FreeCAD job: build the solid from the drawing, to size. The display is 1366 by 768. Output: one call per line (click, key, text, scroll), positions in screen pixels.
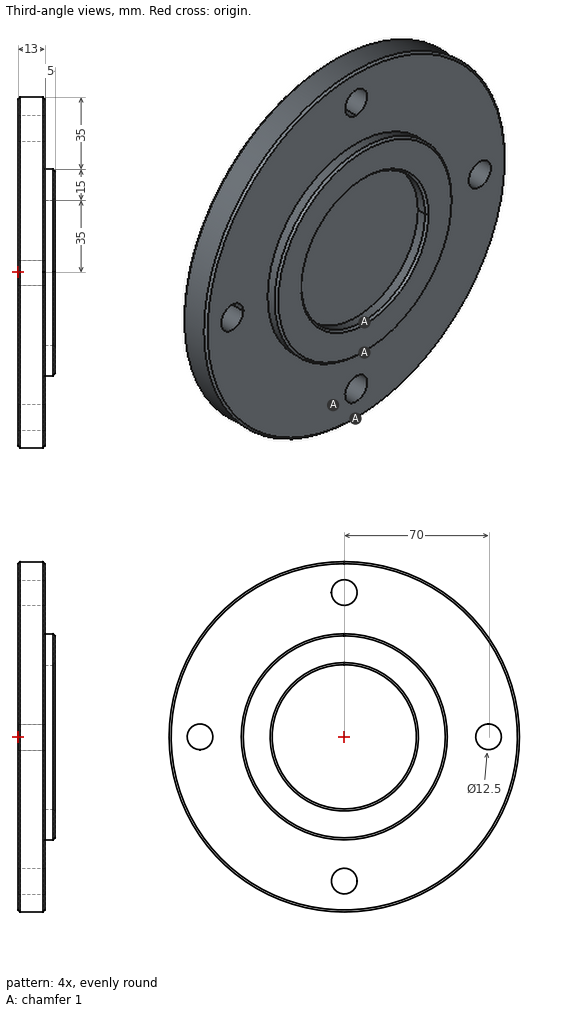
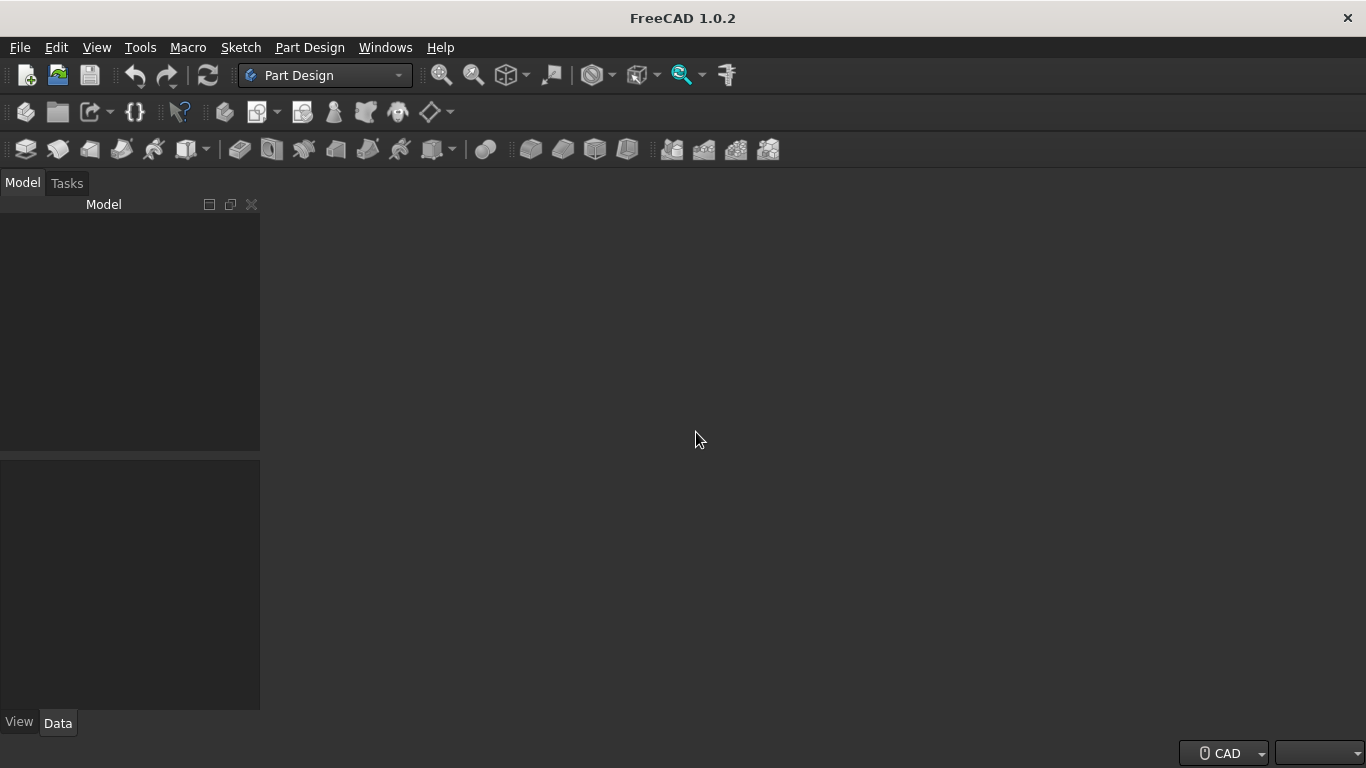
click(26, 76)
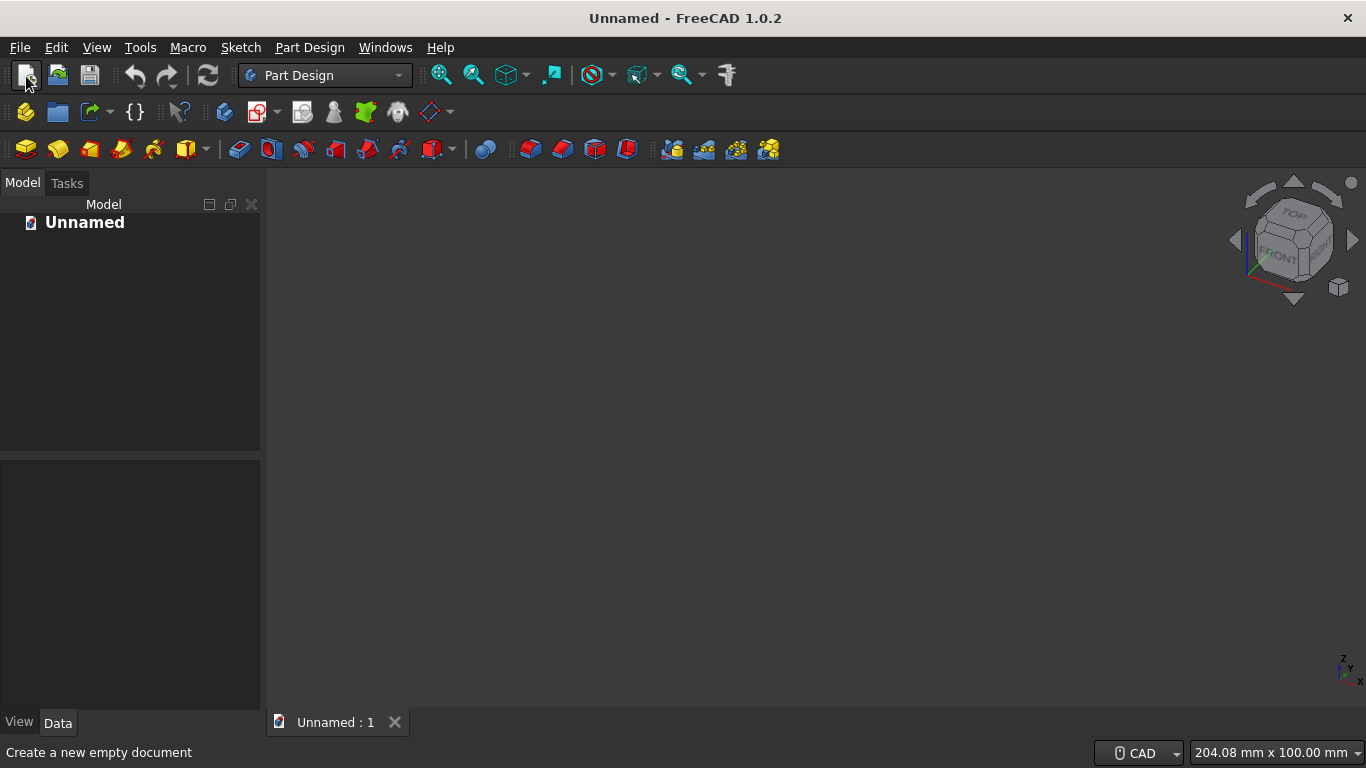
click(258, 112)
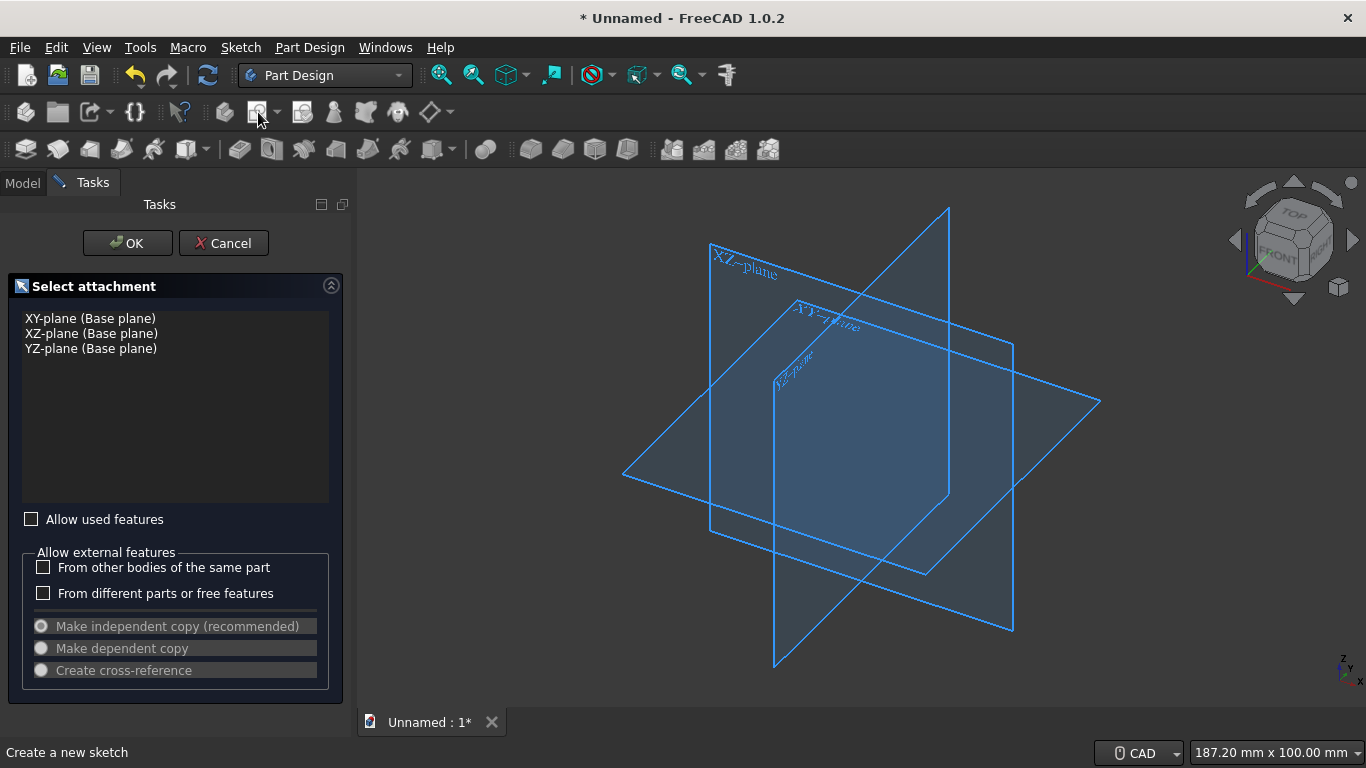
click(82, 318)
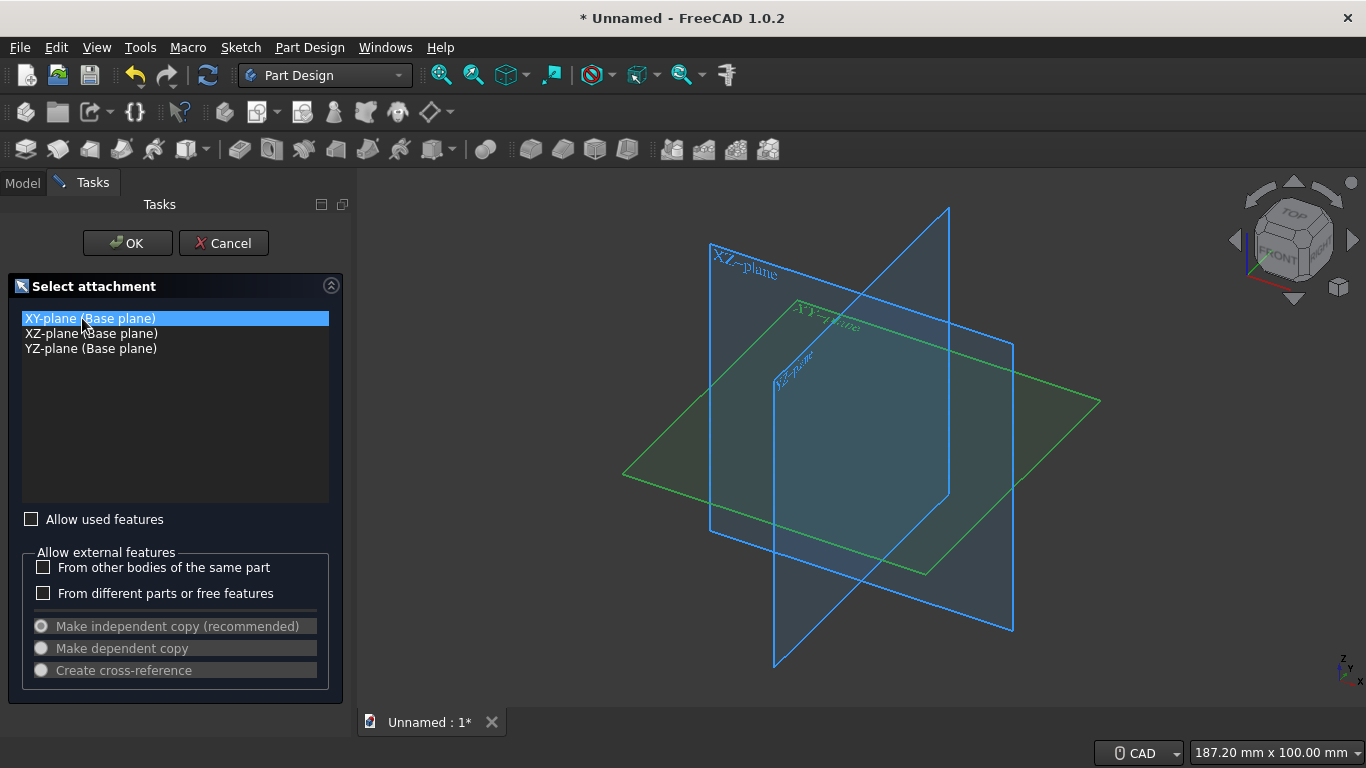
click(128, 243)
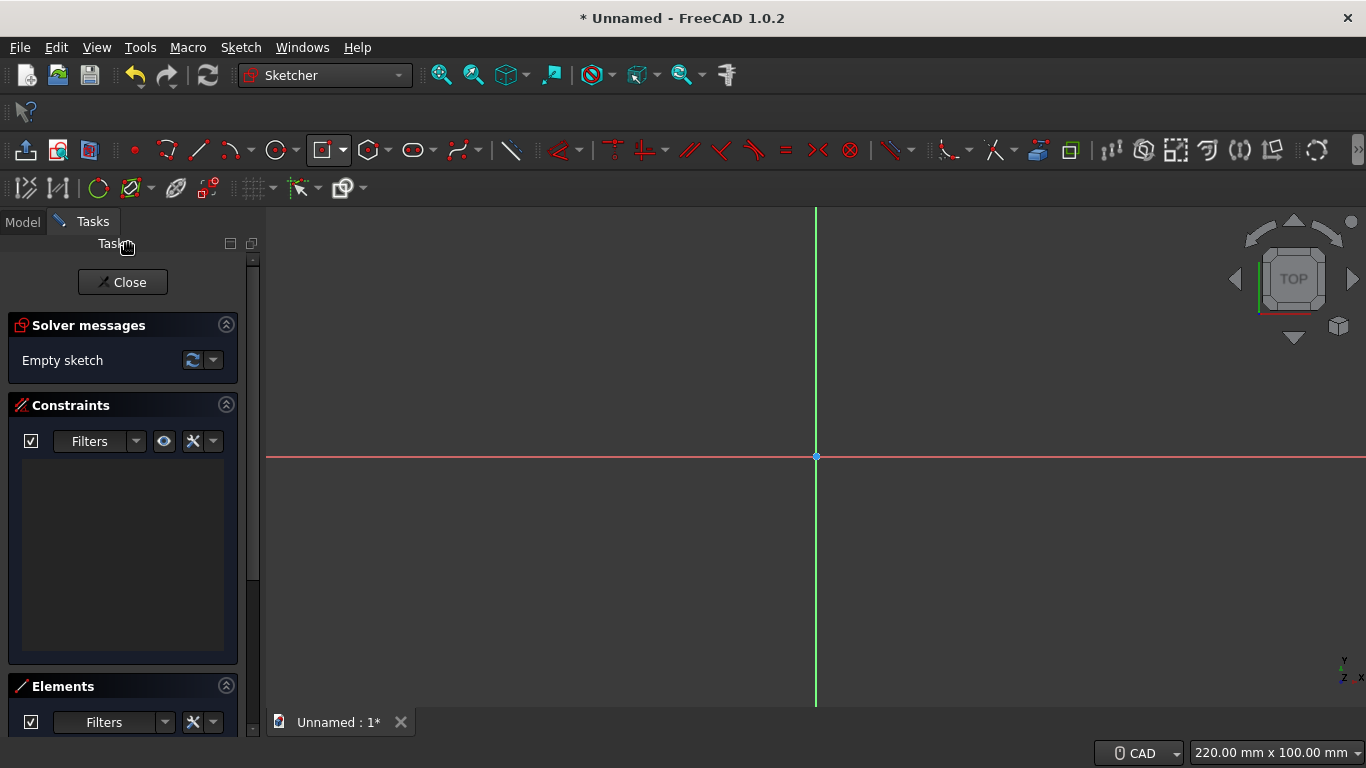
scroll(609, 679, down, 3)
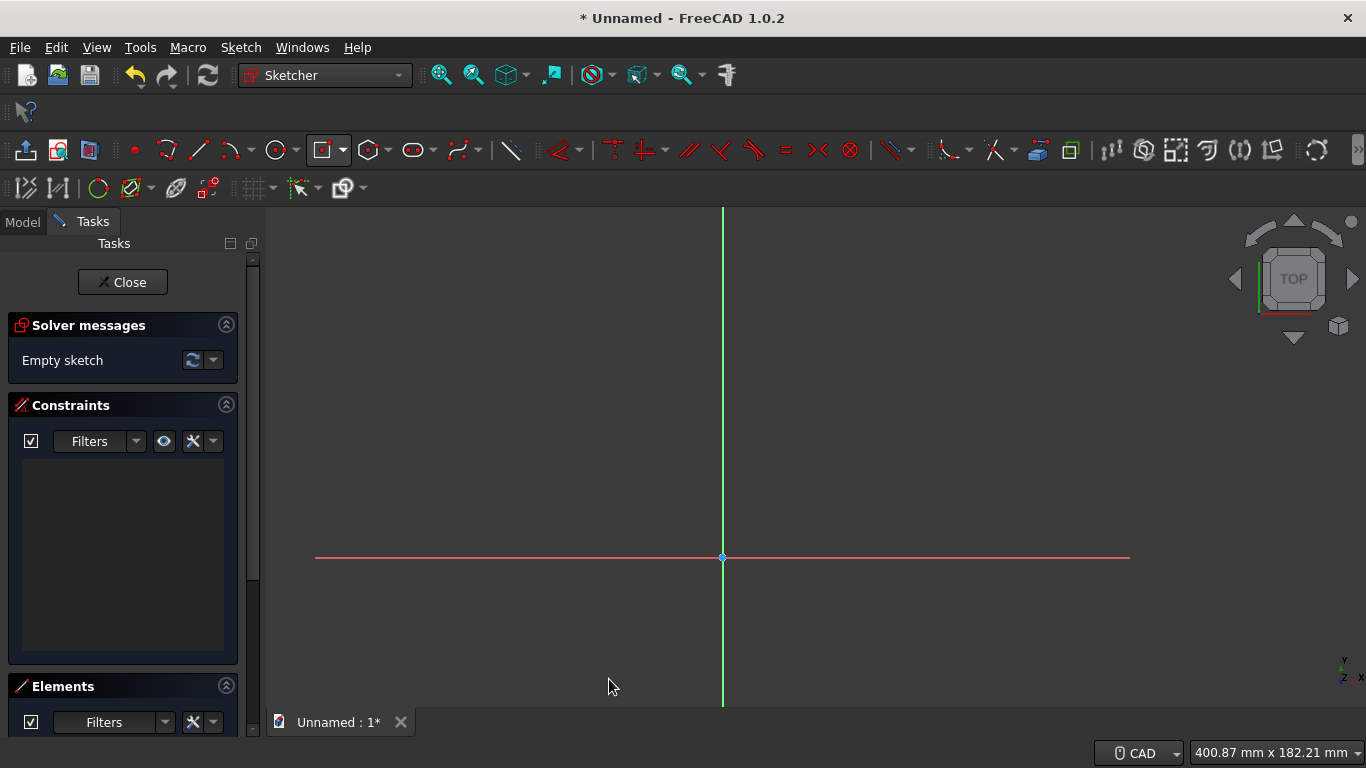
click(168, 150)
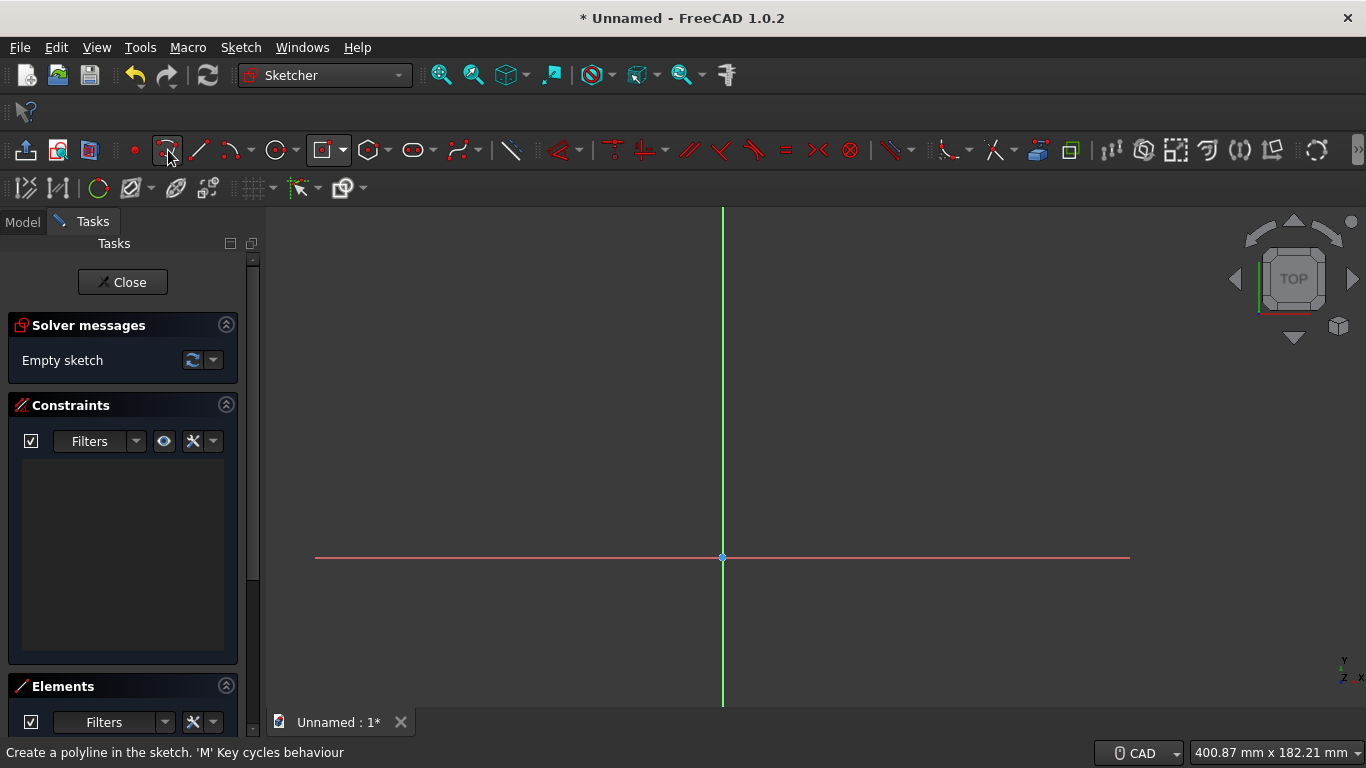
click(723, 558)
click(758, 549)
click(758, 462)
click(772, 462)
click(772, 420)
click(758, 420)
click(758, 324)
click(732, 324)
click(723, 558)
key(Escape)
key(Escape)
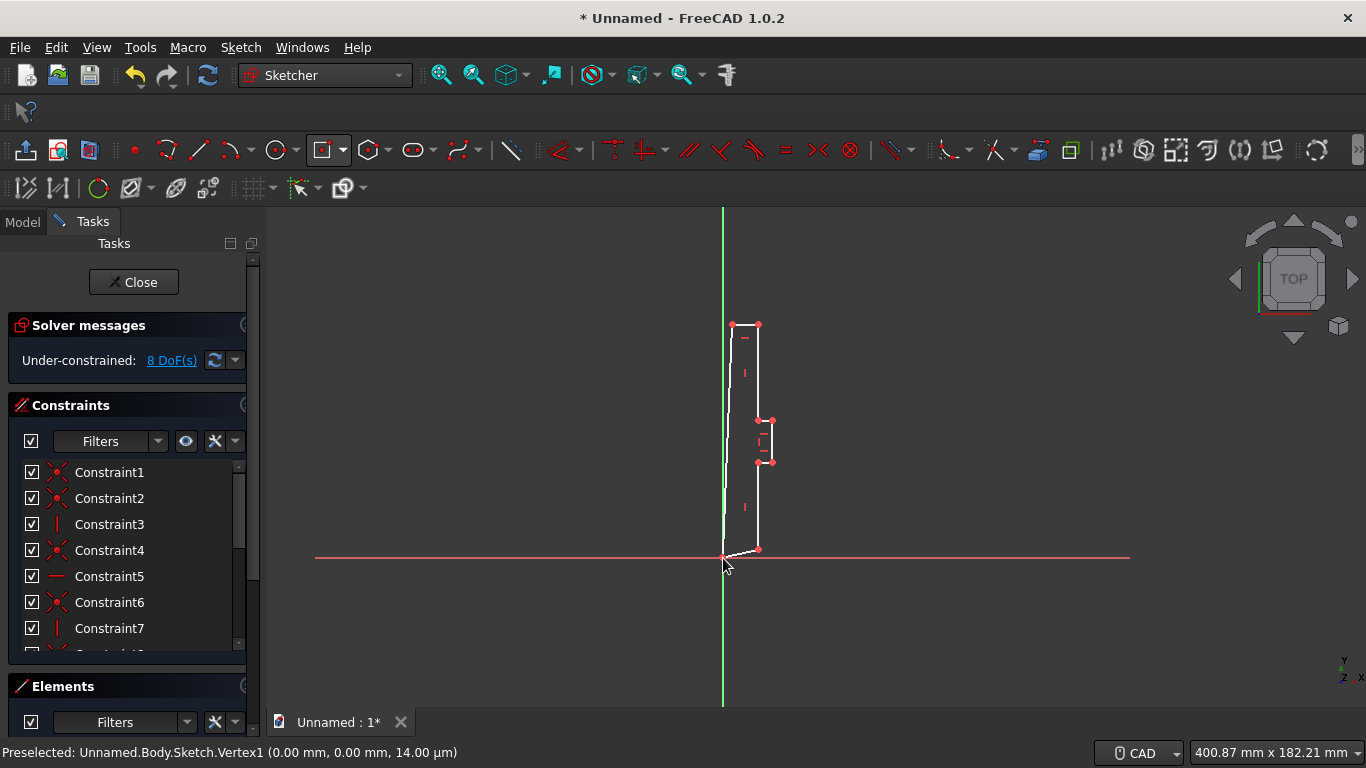
scroll(733, 555, up, 2)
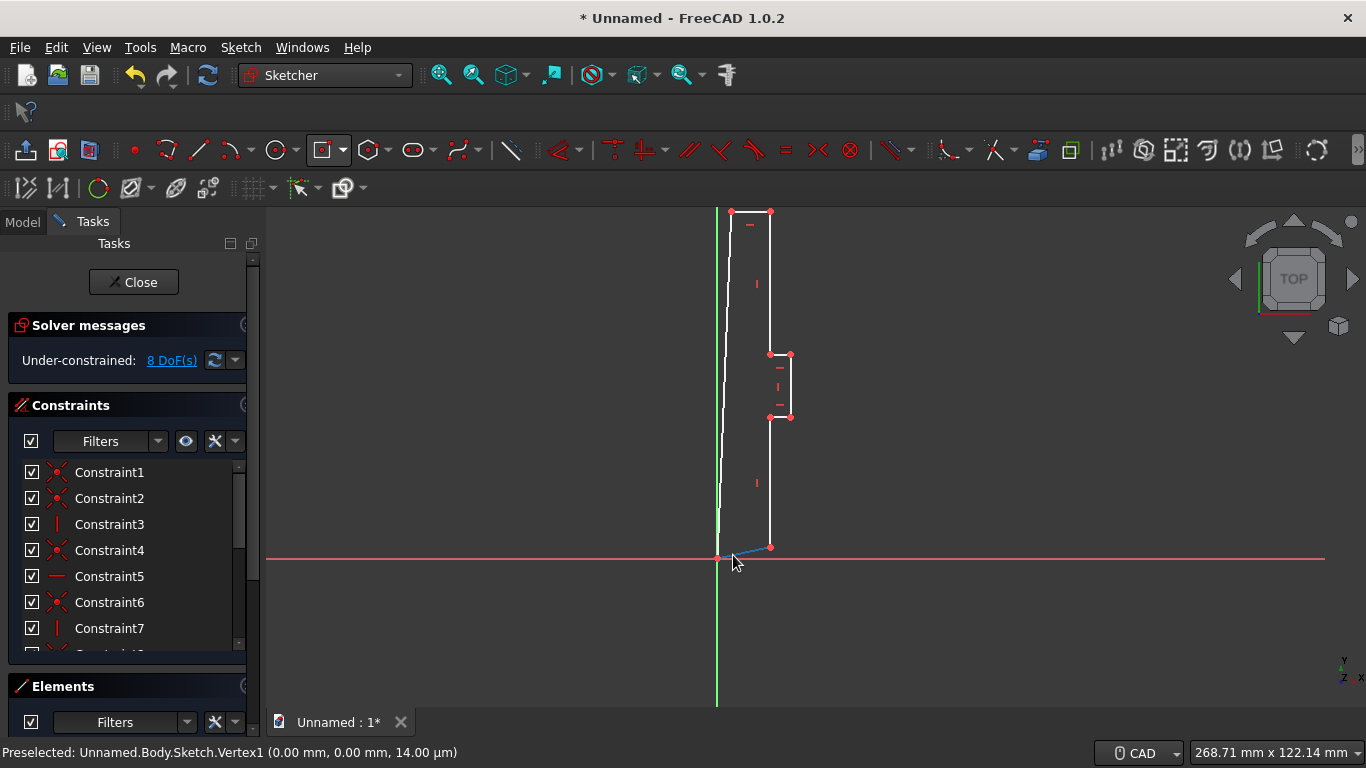
click(733, 555)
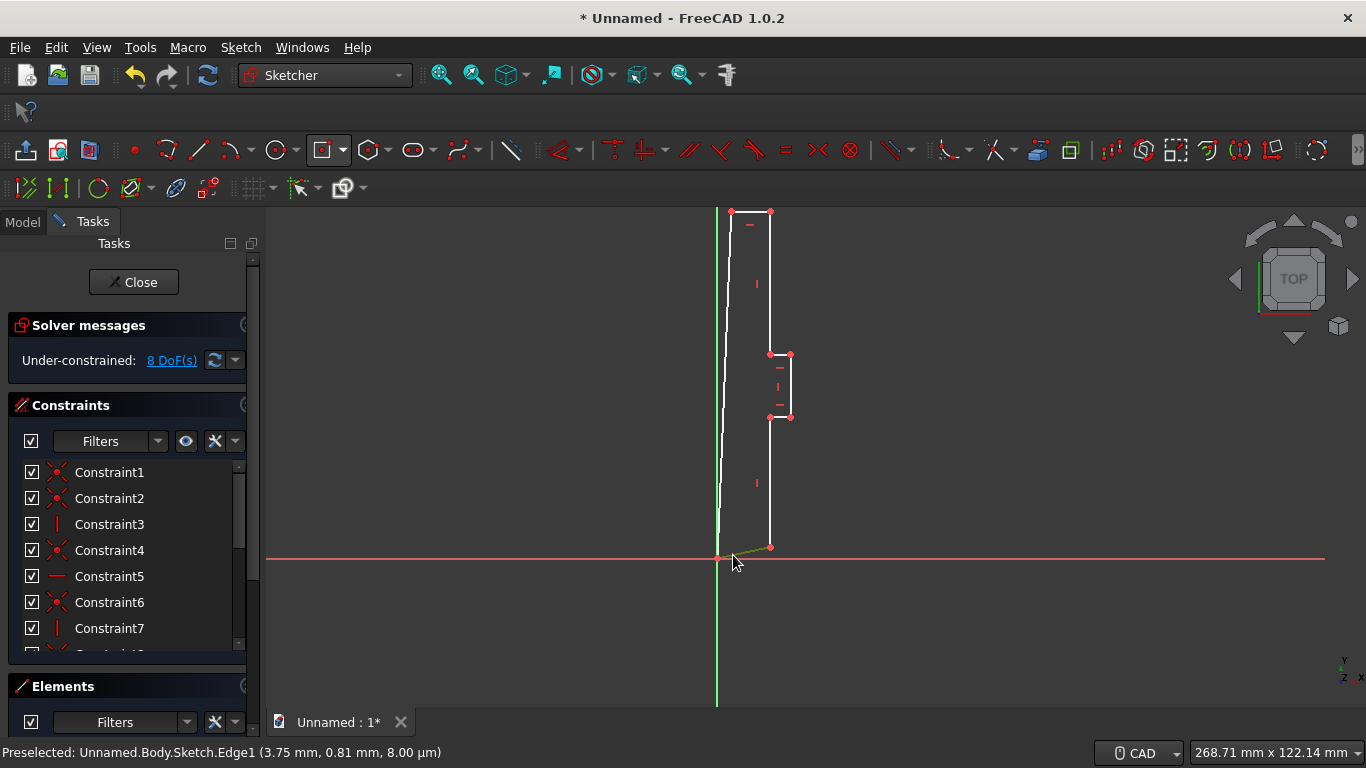
key(h)